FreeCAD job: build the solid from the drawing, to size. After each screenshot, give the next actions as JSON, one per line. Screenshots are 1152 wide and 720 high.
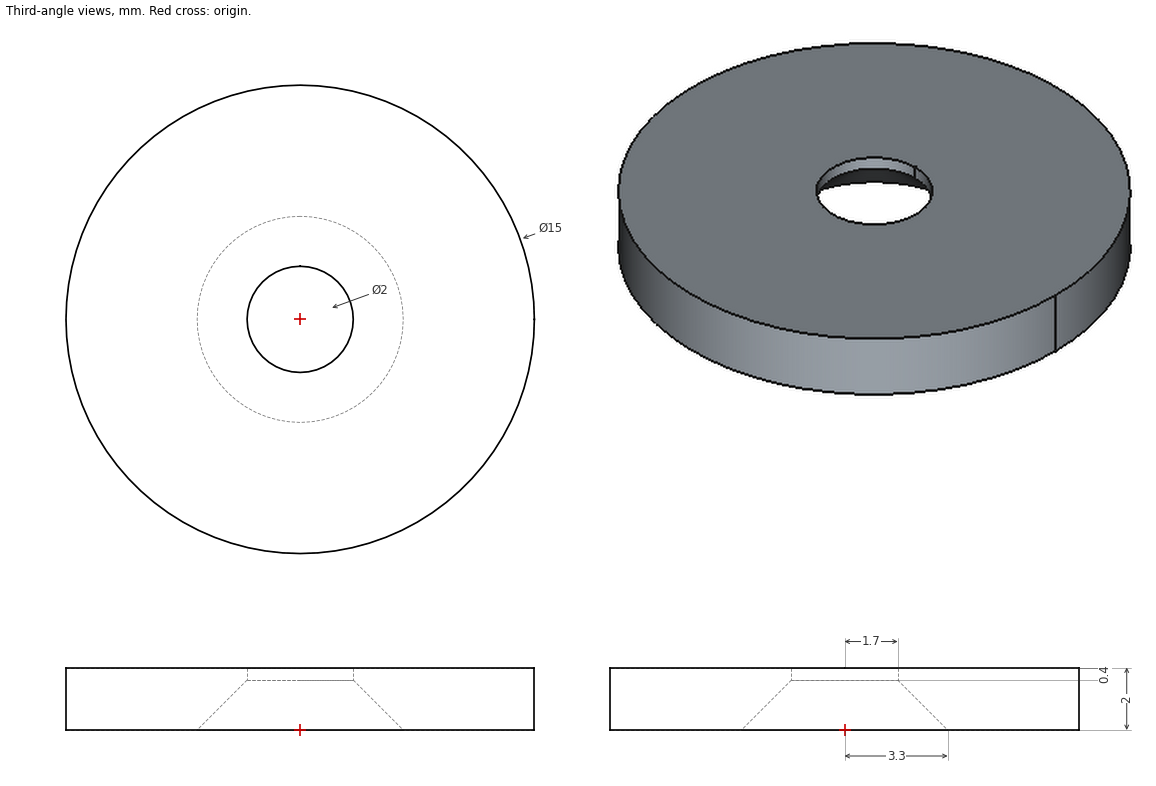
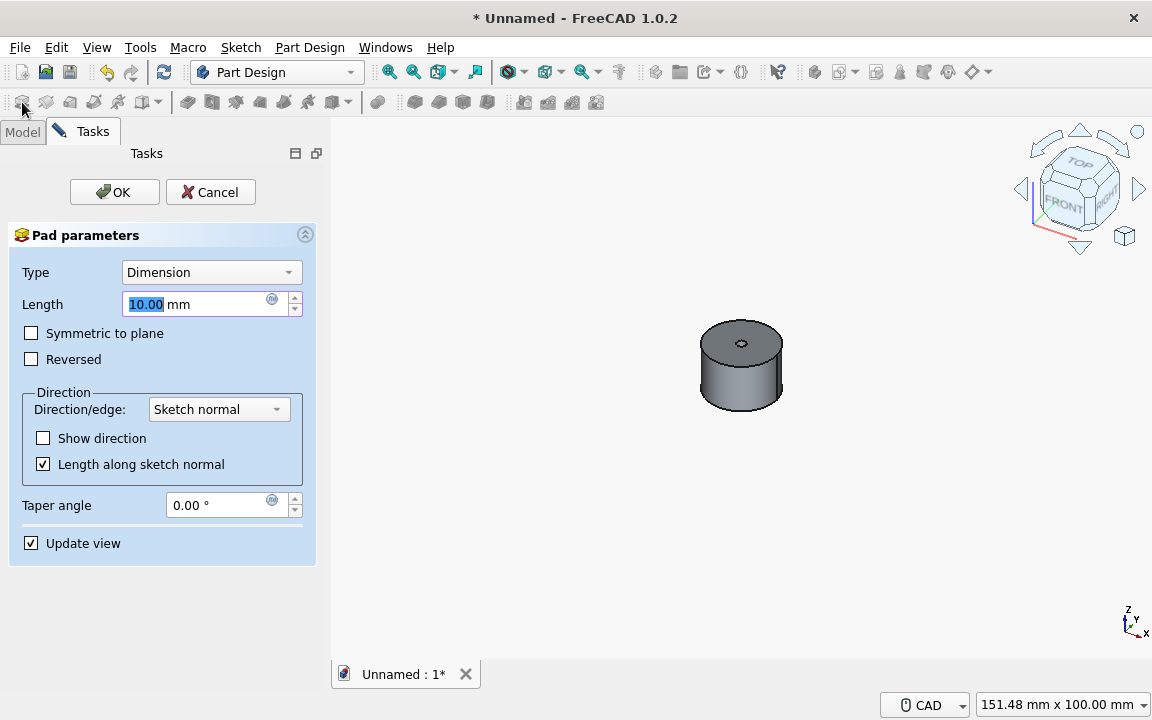
{"action": "type", "text": "2"}
{"action": "key", "text": "Tab"}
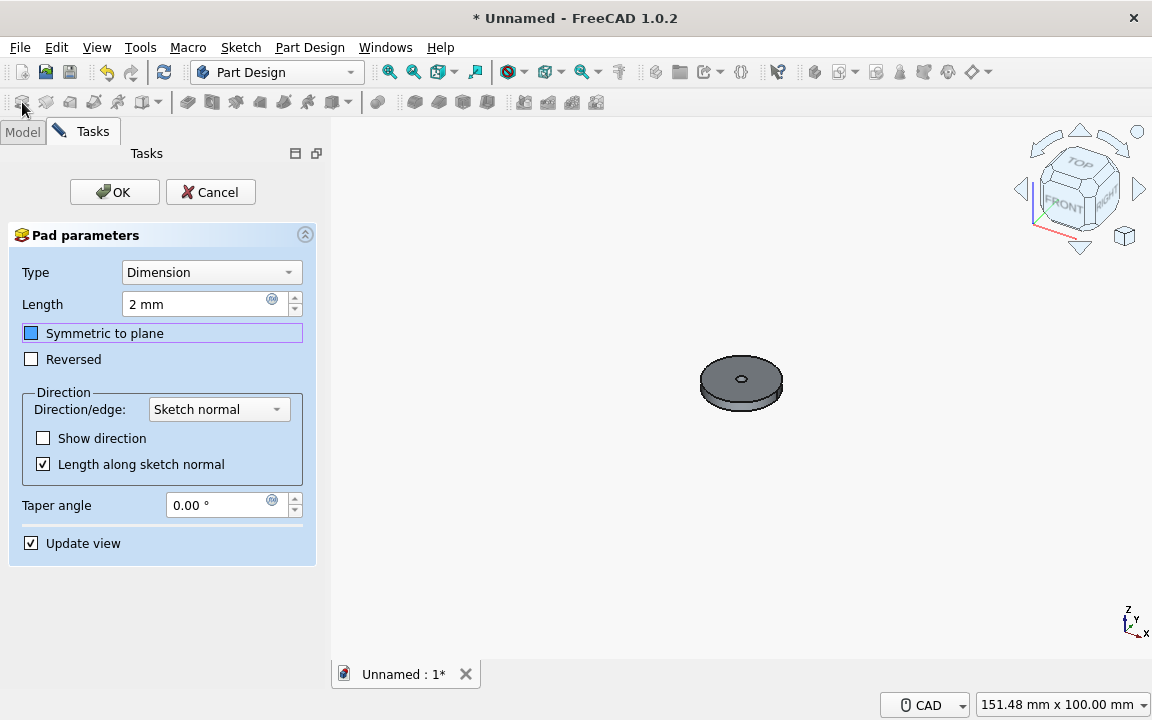
{"action": "left_click", "coordinate": [115, 192]}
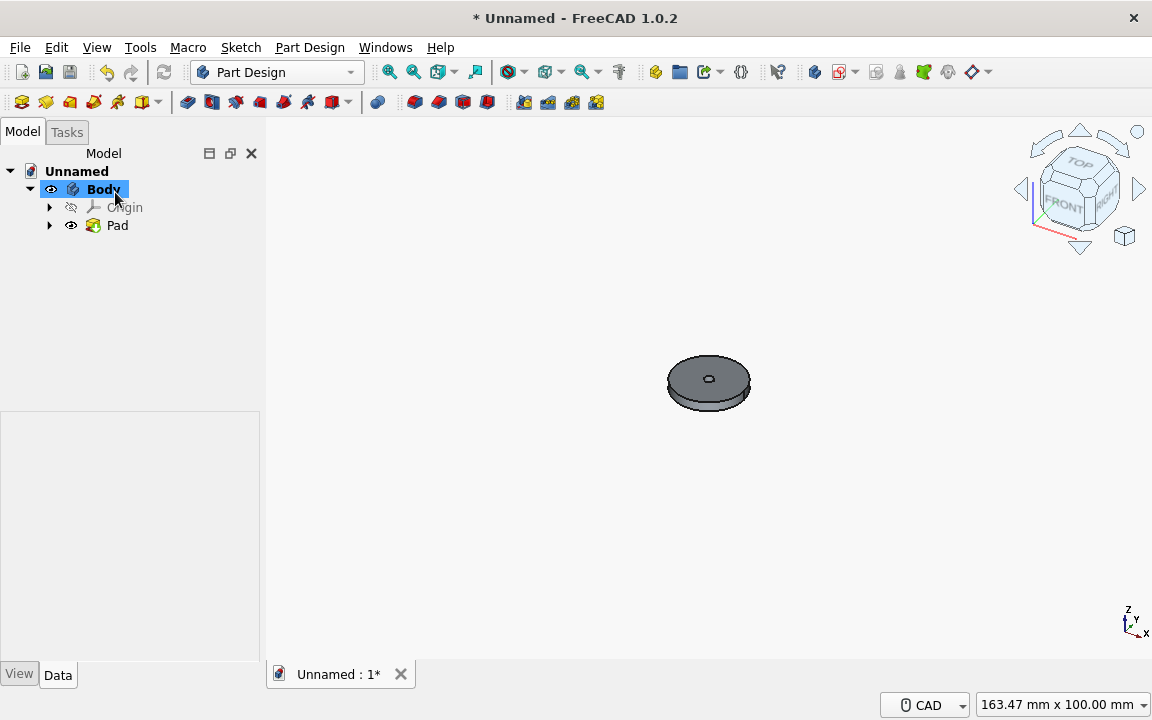
{"action": "left_click", "coordinate": [390, 72]}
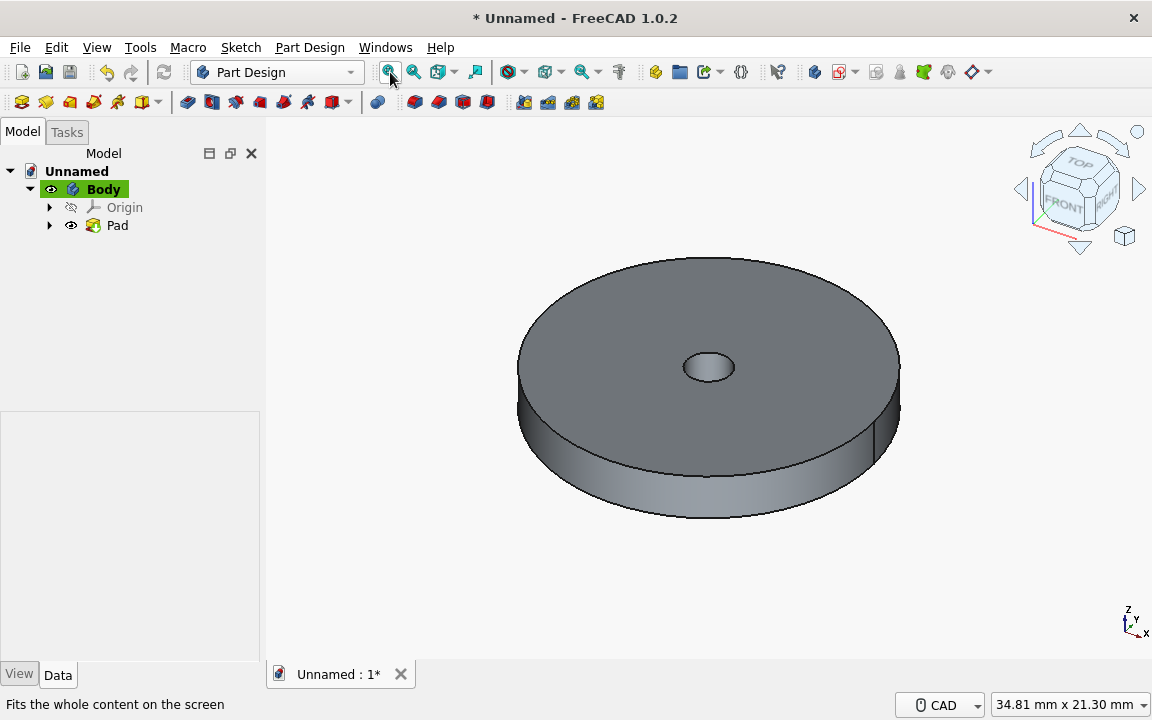
{"action": "left_click", "coordinate": [840, 72]}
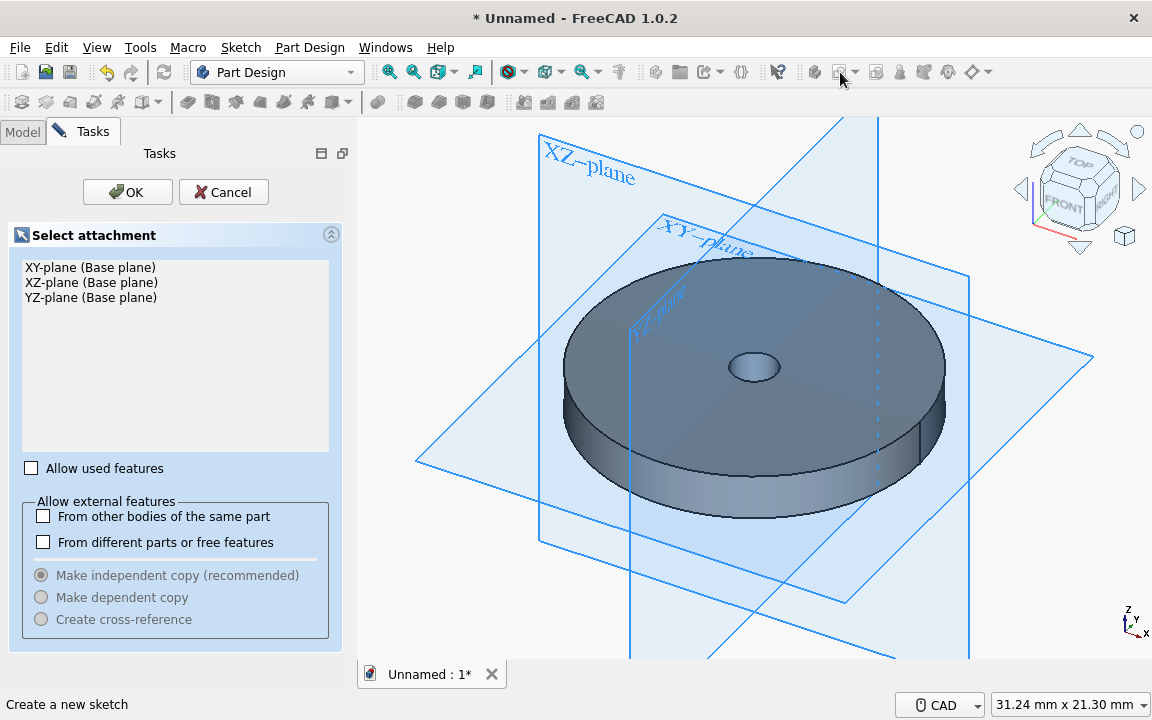
{"action": "left_click", "coordinate": [82, 298]}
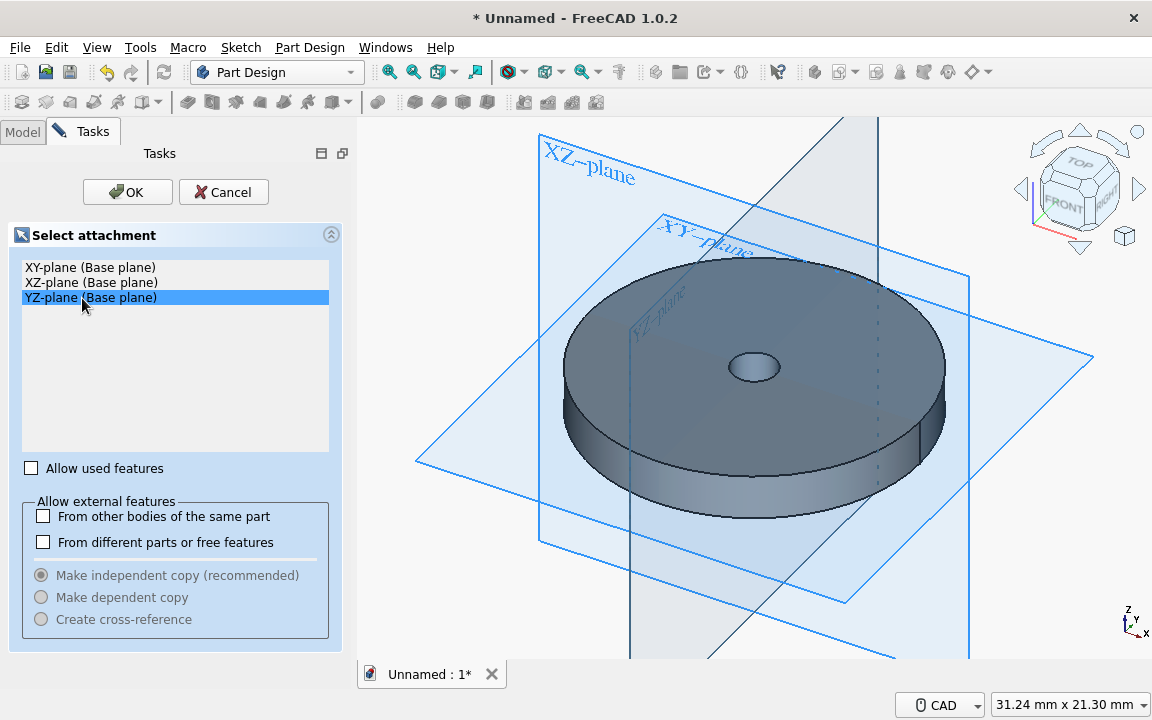
{"action": "left_click", "coordinate": [128, 192]}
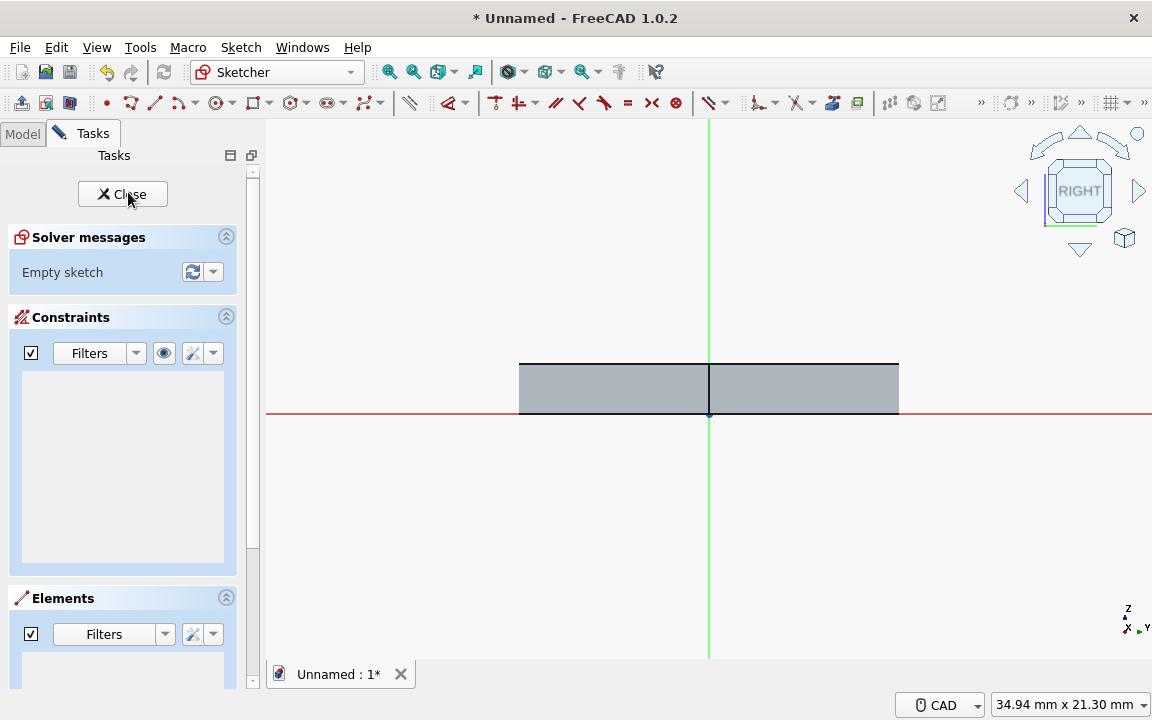
{"action": "left_click", "coordinate": [70, 104]}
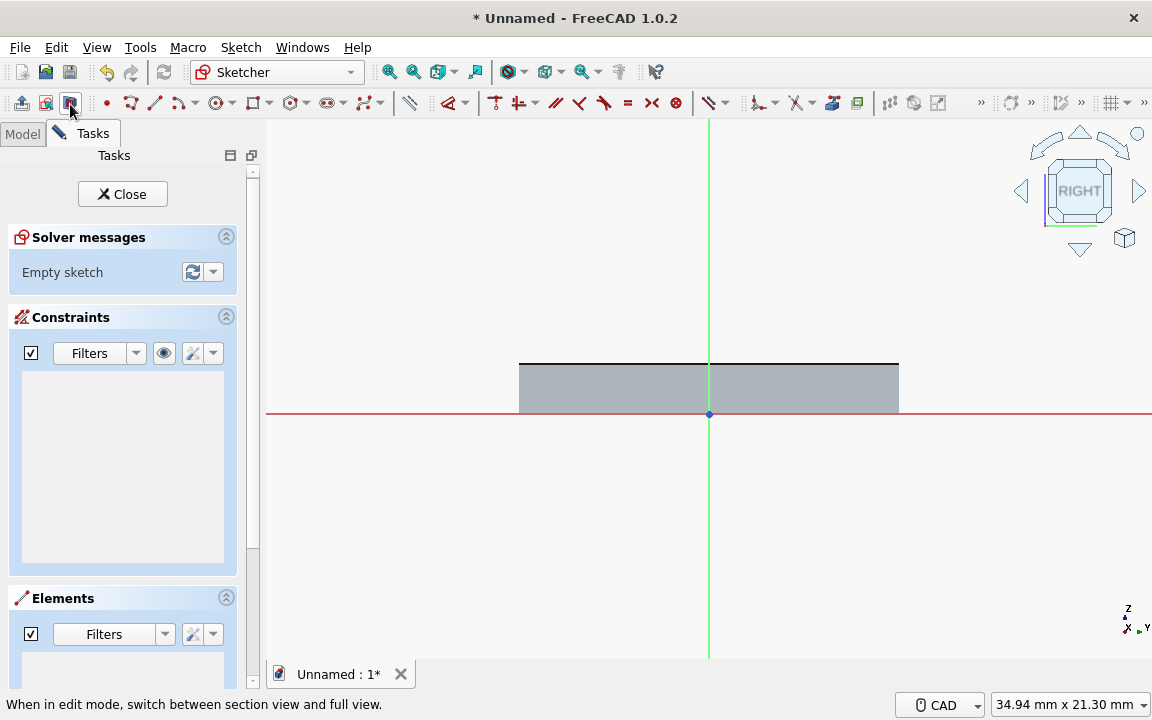
{"action": "scroll", "coordinate": [773, 389], "scroll_direction": "up", "scroll_amount": 9}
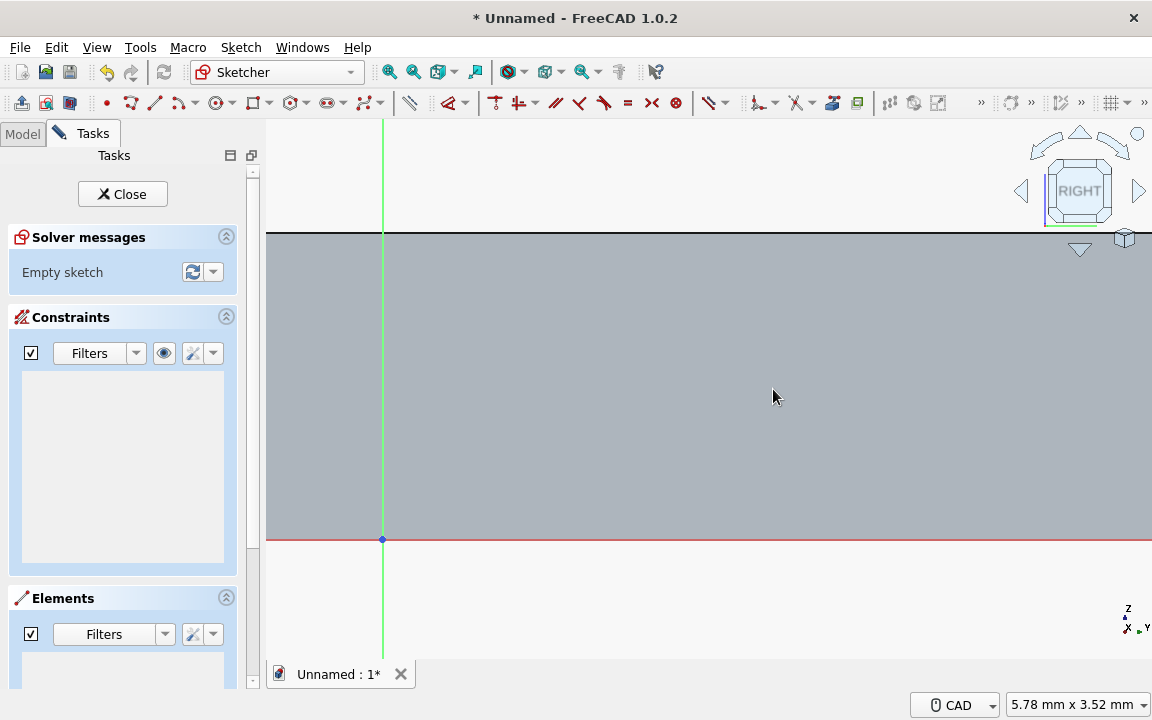
{"action": "left_click", "coordinate": [132, 104]}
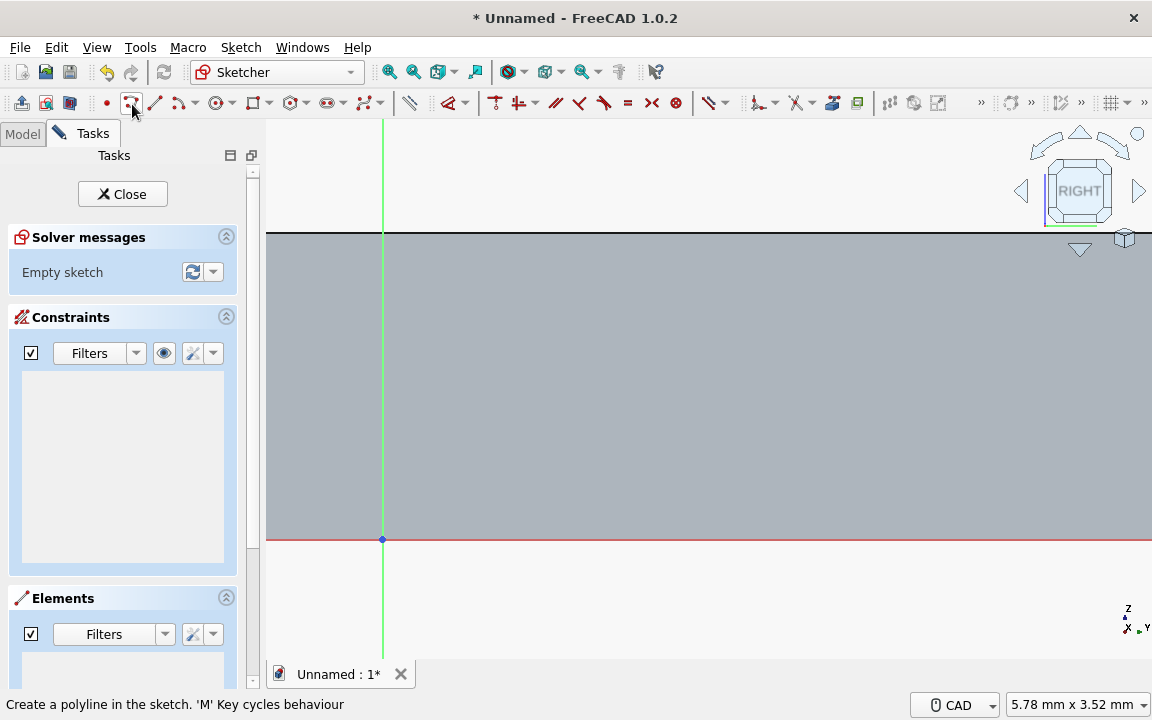
{"action": "left_click", "coordinate": [383, 540]}
{"action": "left_click", "coordinate": [889, 531]}
{"action": "left_click", "coordinate": [644, 294]}
{"action": "left_click", "coordinate": [644, 233]}
{"action": "left_click", "coordinate": [392, 233]}
{"action": "left_click", "coordinate": [383, 540]}
{"action": "key", "text": "Escape"}
{"action": "key", "text": "Escape"}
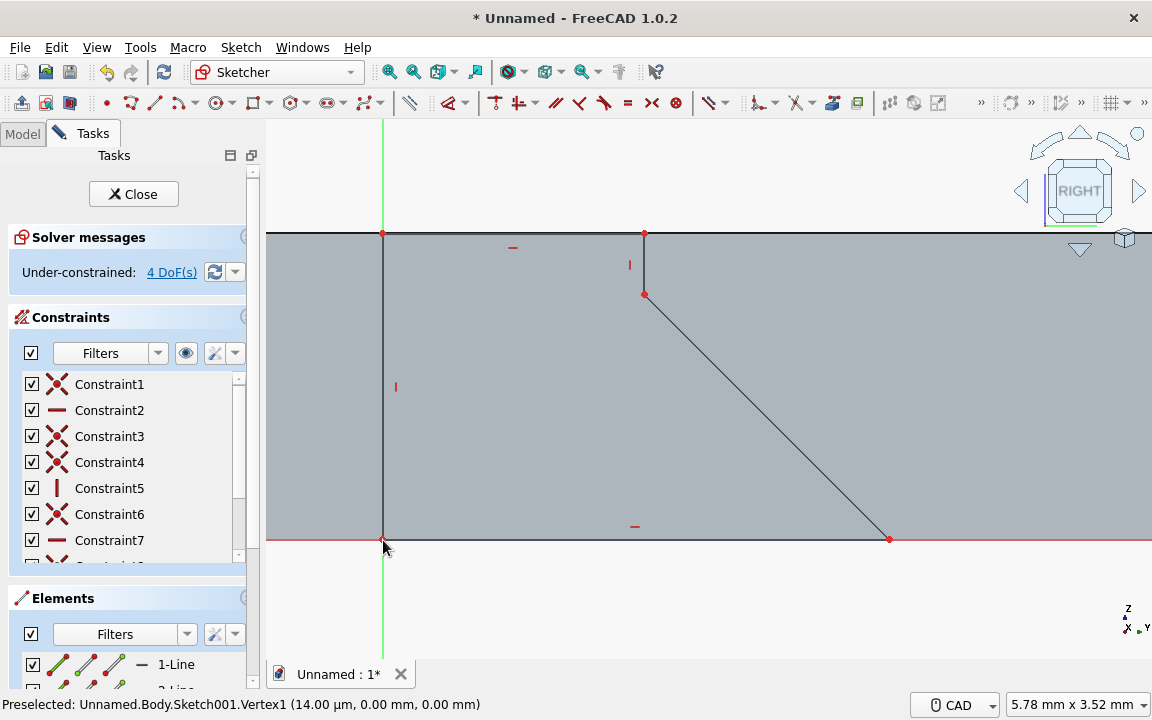
{"action": "left_click", "coordinate": [448, 104]}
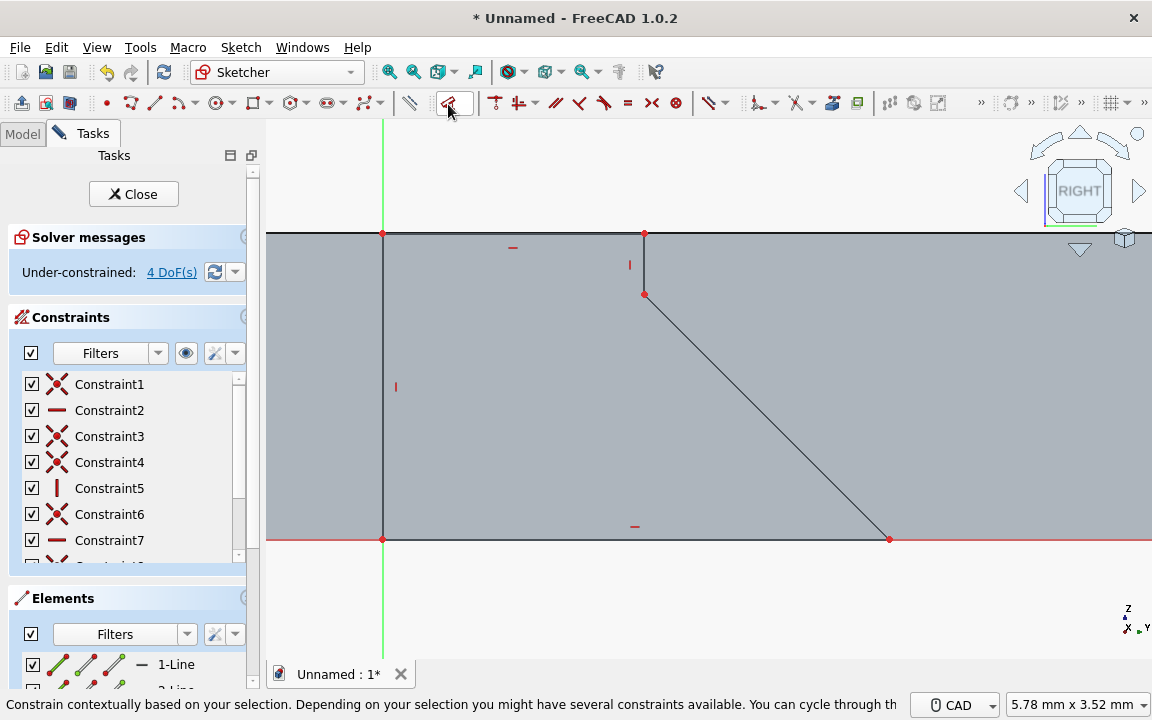
{"action": "left_click", "coordinate": [383, 326]}
{"action": "left_click", "coordinate": [349, 387]}